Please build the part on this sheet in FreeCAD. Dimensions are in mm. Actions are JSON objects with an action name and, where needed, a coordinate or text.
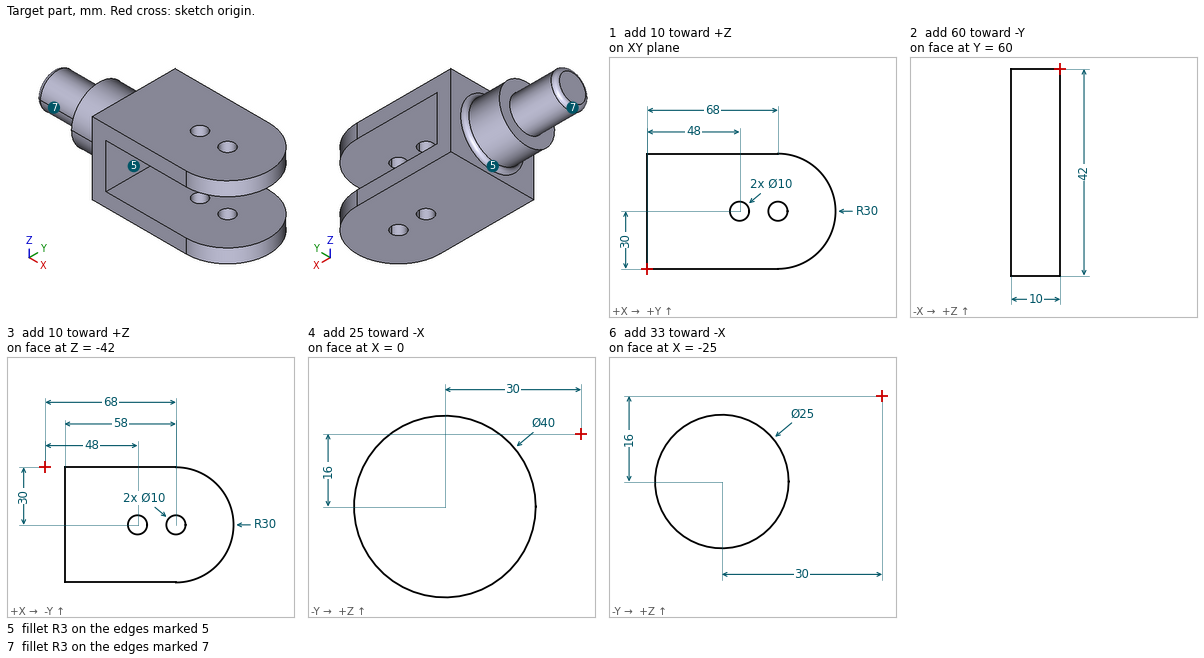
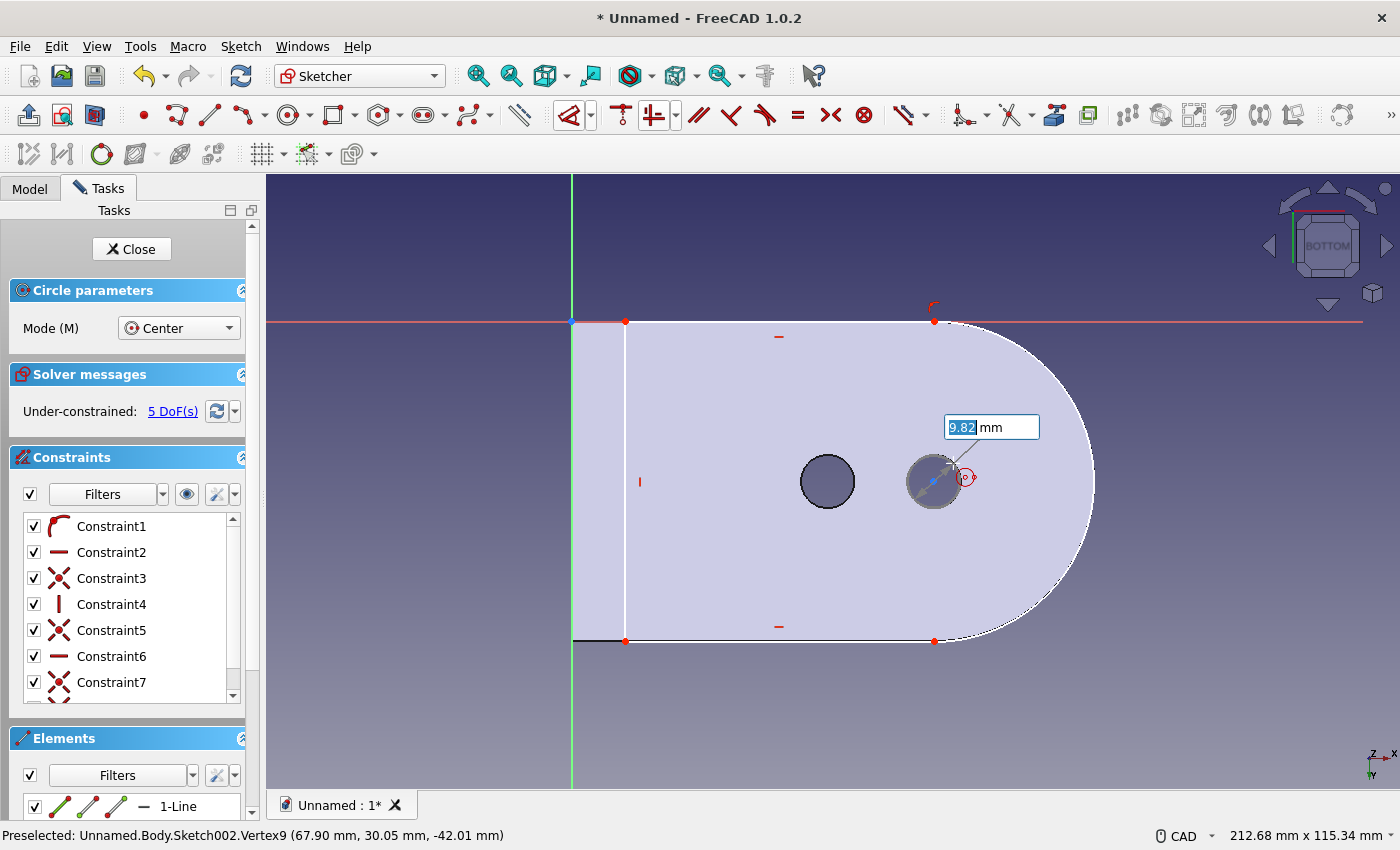
{"action": "type", "text": "10"}
{"action": "key", "text": "Return"}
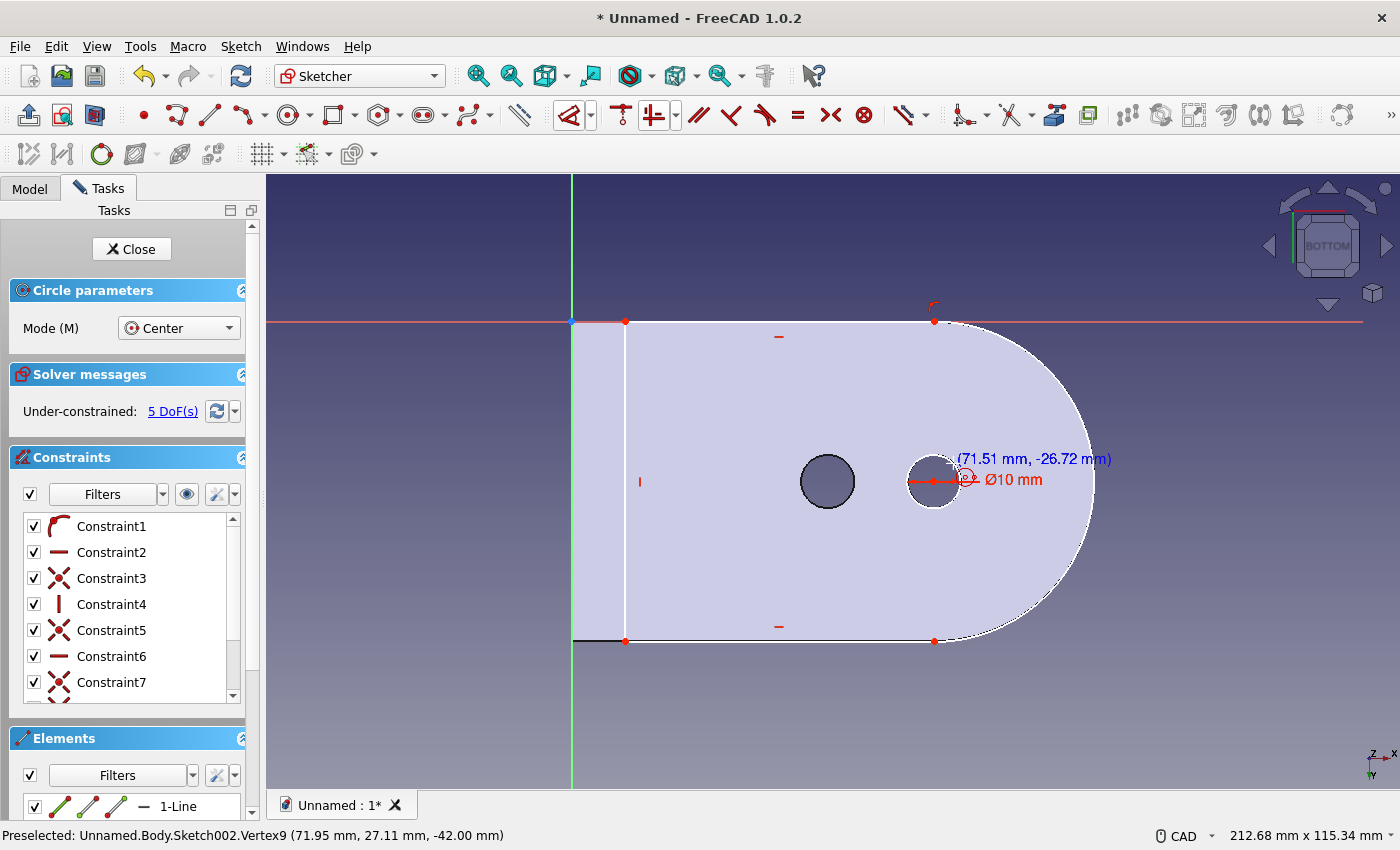
{"action": "left_click", "coordinate": [828, 482]}
{"action": "mouse_move", "coordinate": [847, 463]}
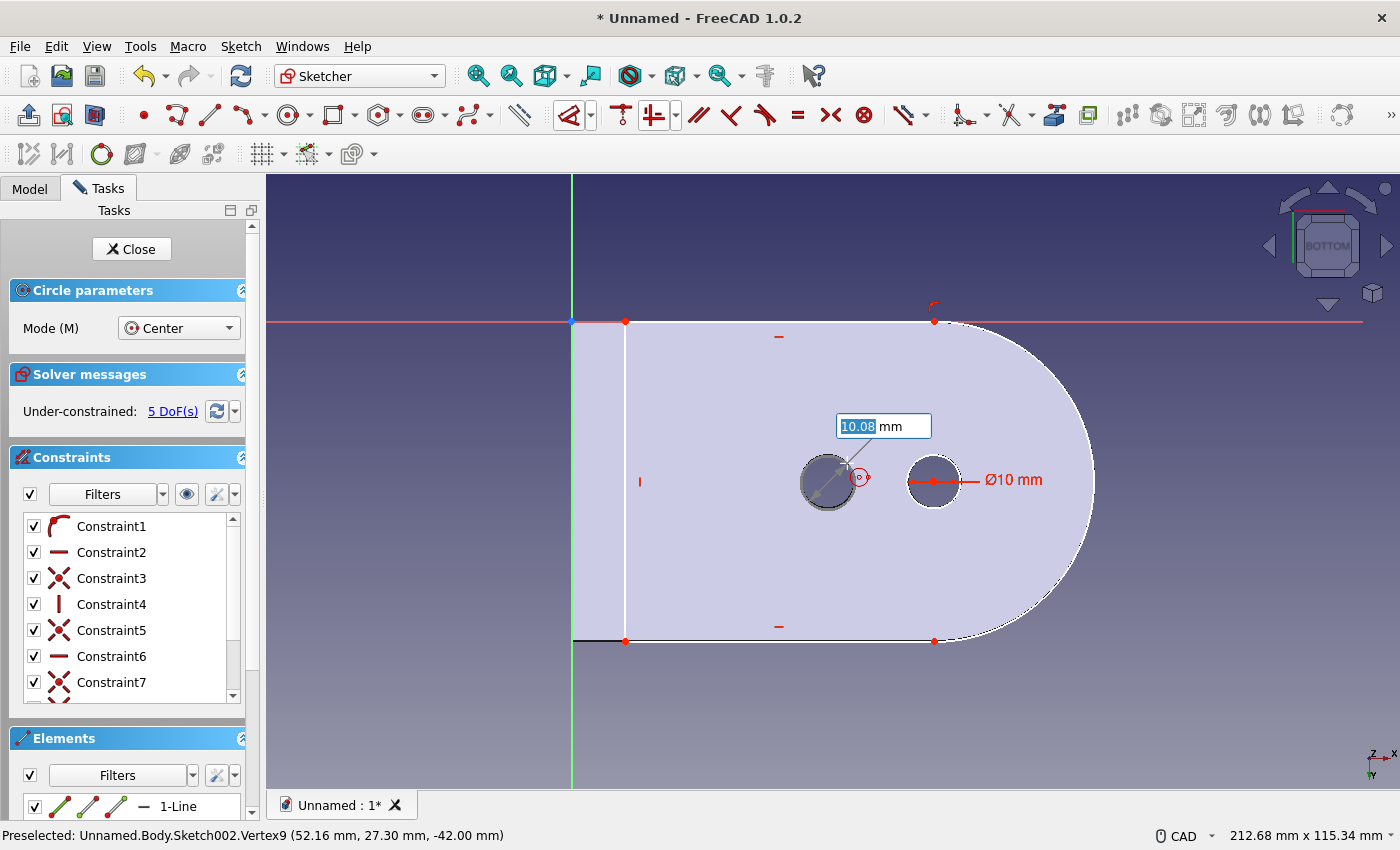
{"action": "type", "text": "10"}
{"action": "key", "text": "Return"}
{"action": "key", "text": "Escape"}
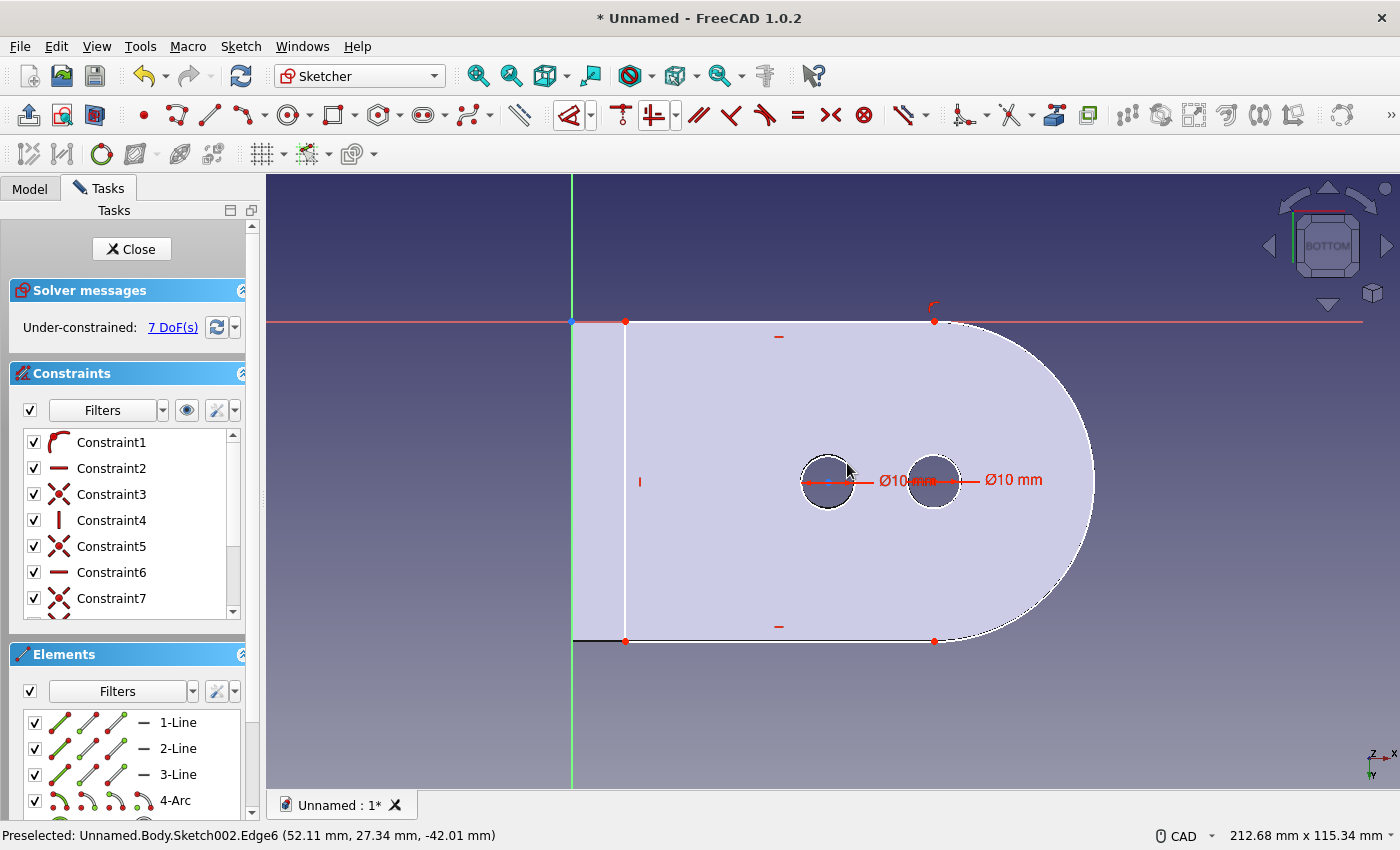
{"action": "left_click", "coordinate": [841, 322]}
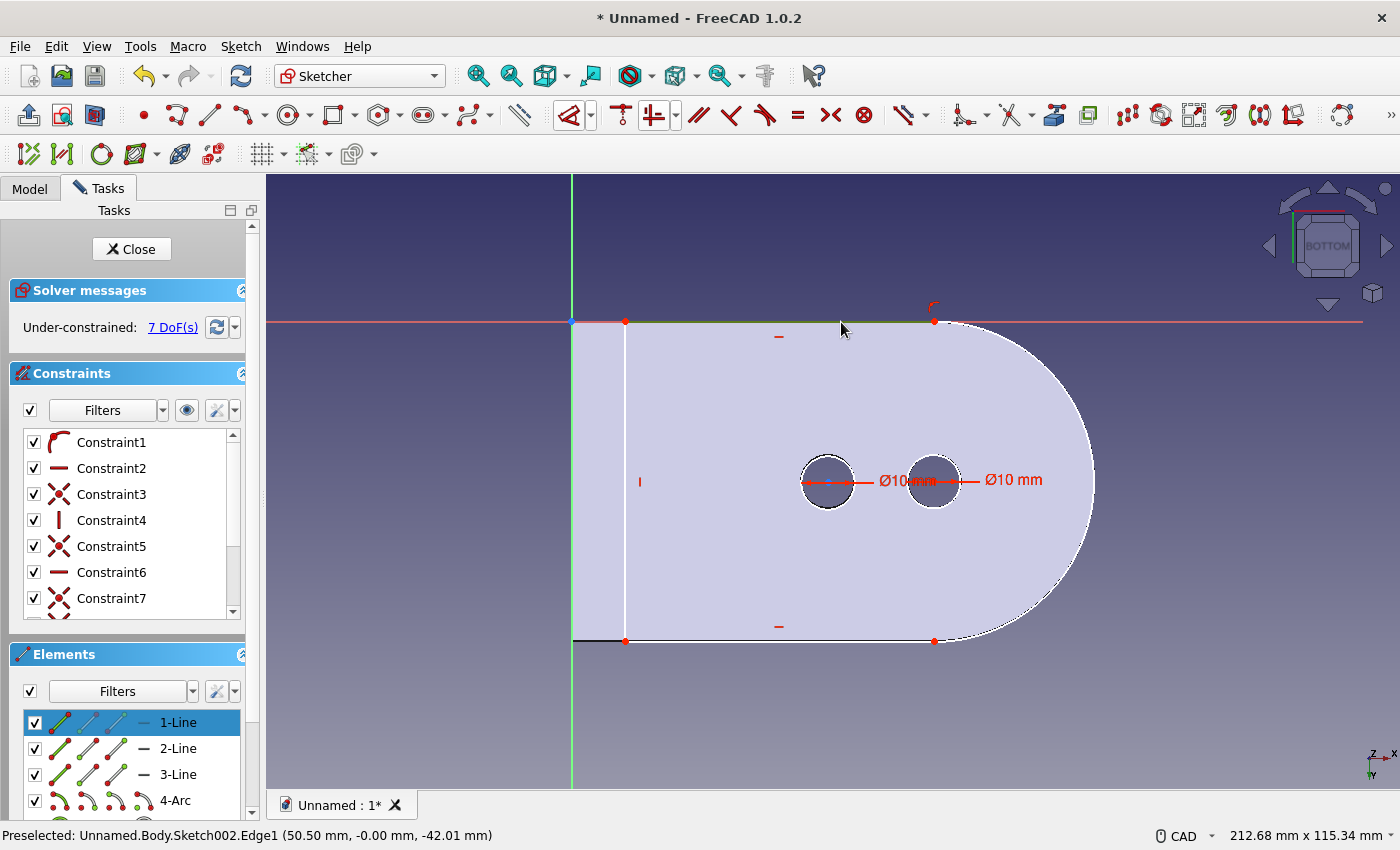
{"action": "left_click", "coordinate": [1063, 576]}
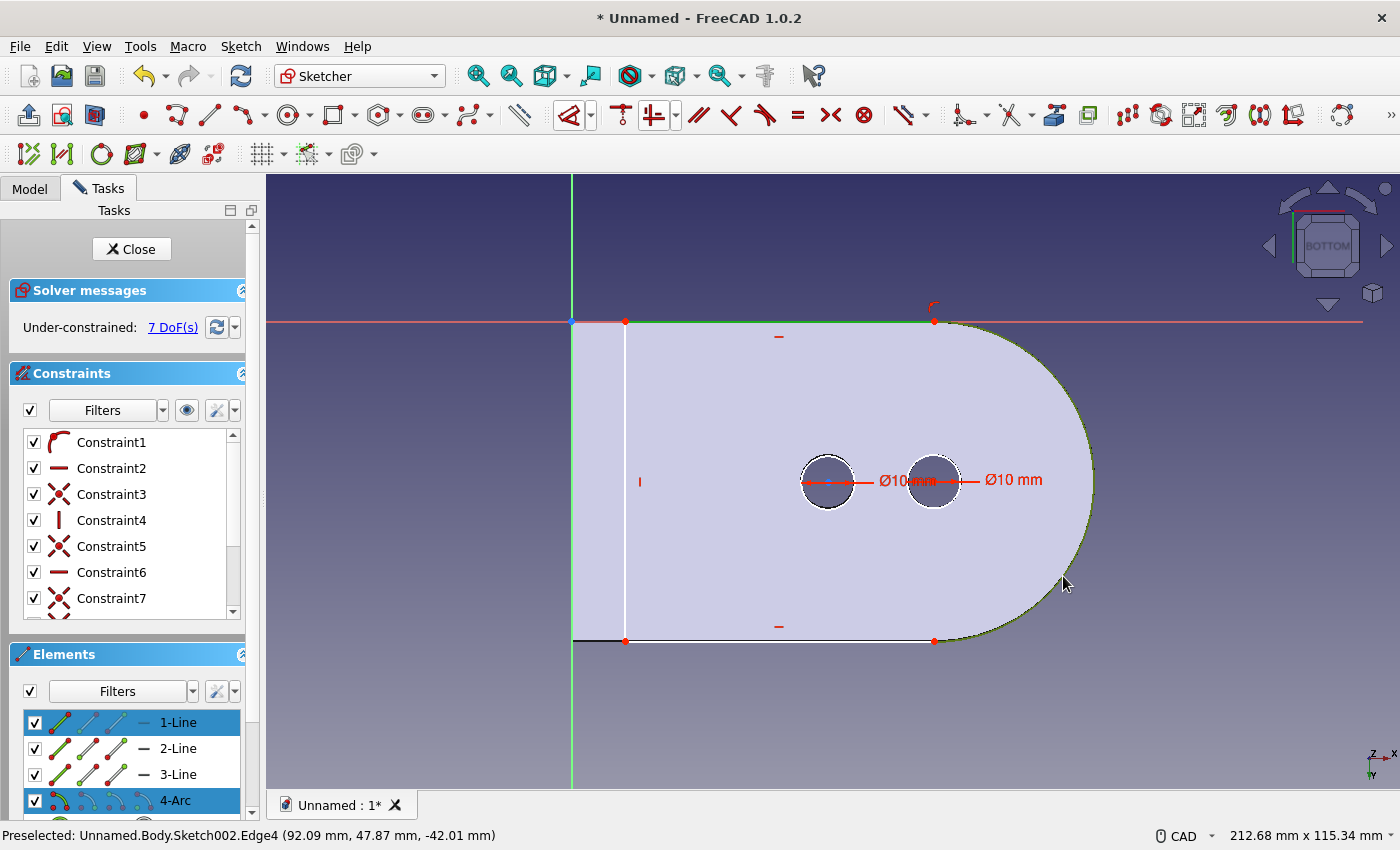
{"action": "left_click", "coordinate": [765, 116]}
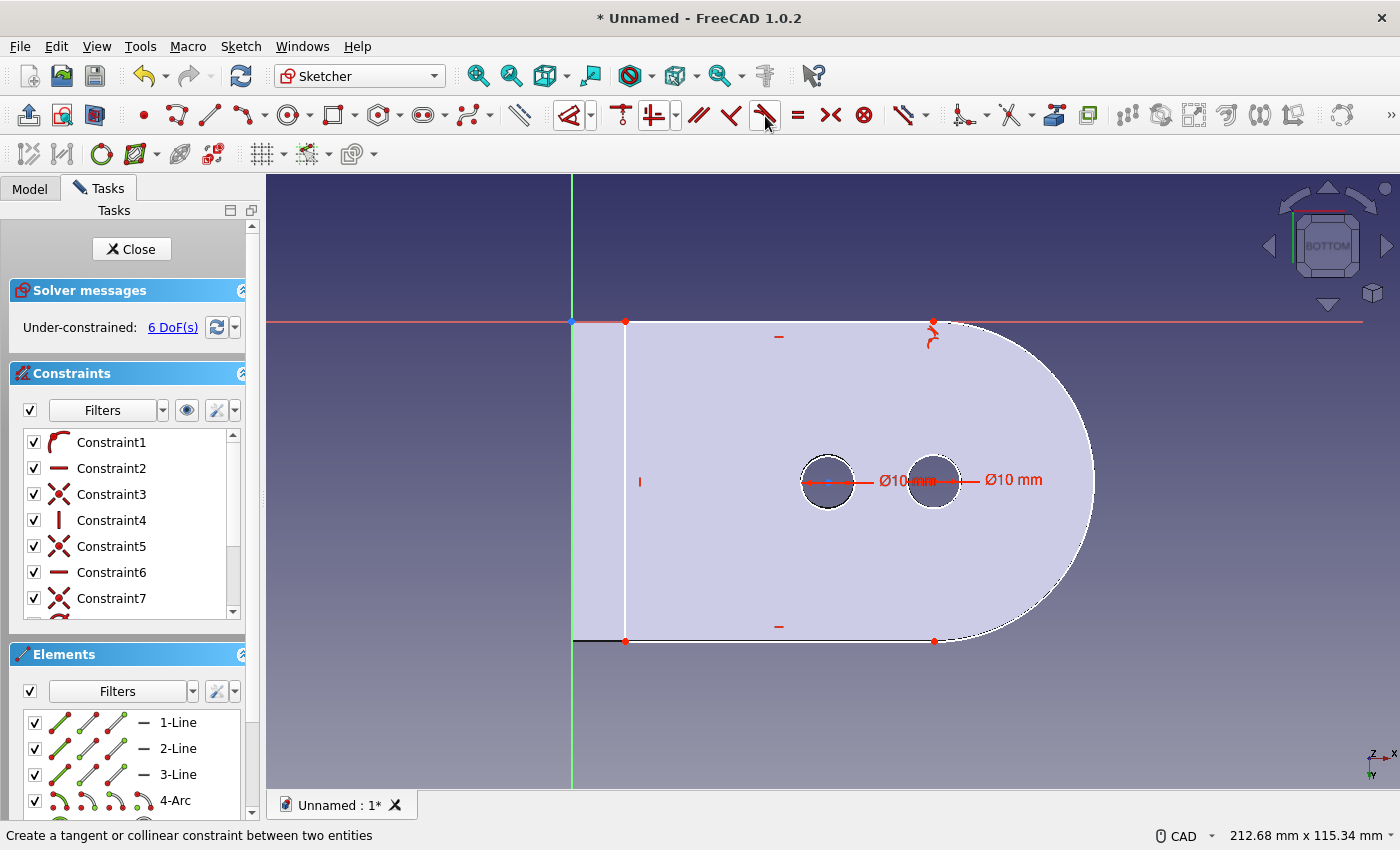
{"action": "left_click", "coordinate": [718, 642]}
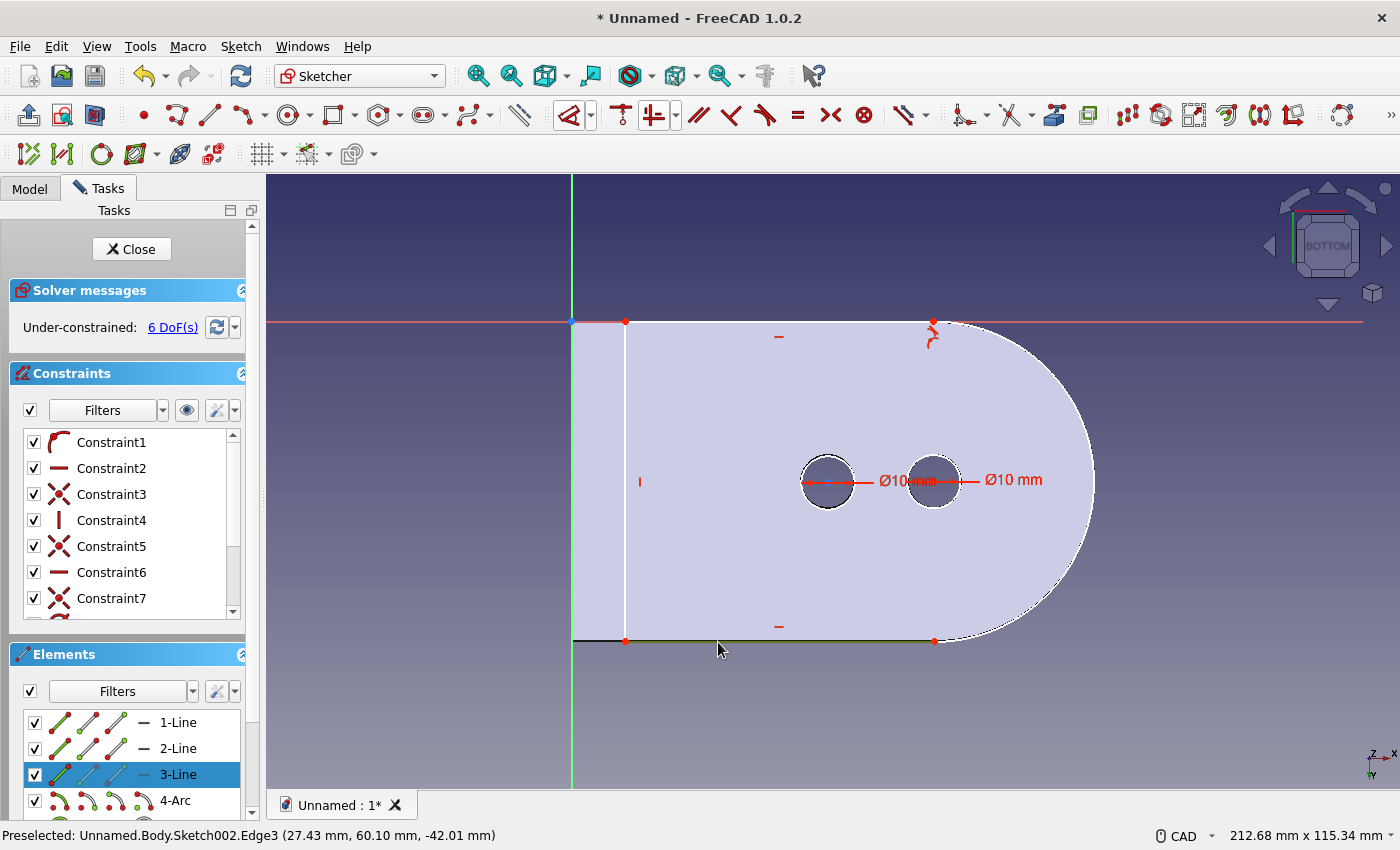
{"action": "left_click", "coordinate": [1063, 576]}